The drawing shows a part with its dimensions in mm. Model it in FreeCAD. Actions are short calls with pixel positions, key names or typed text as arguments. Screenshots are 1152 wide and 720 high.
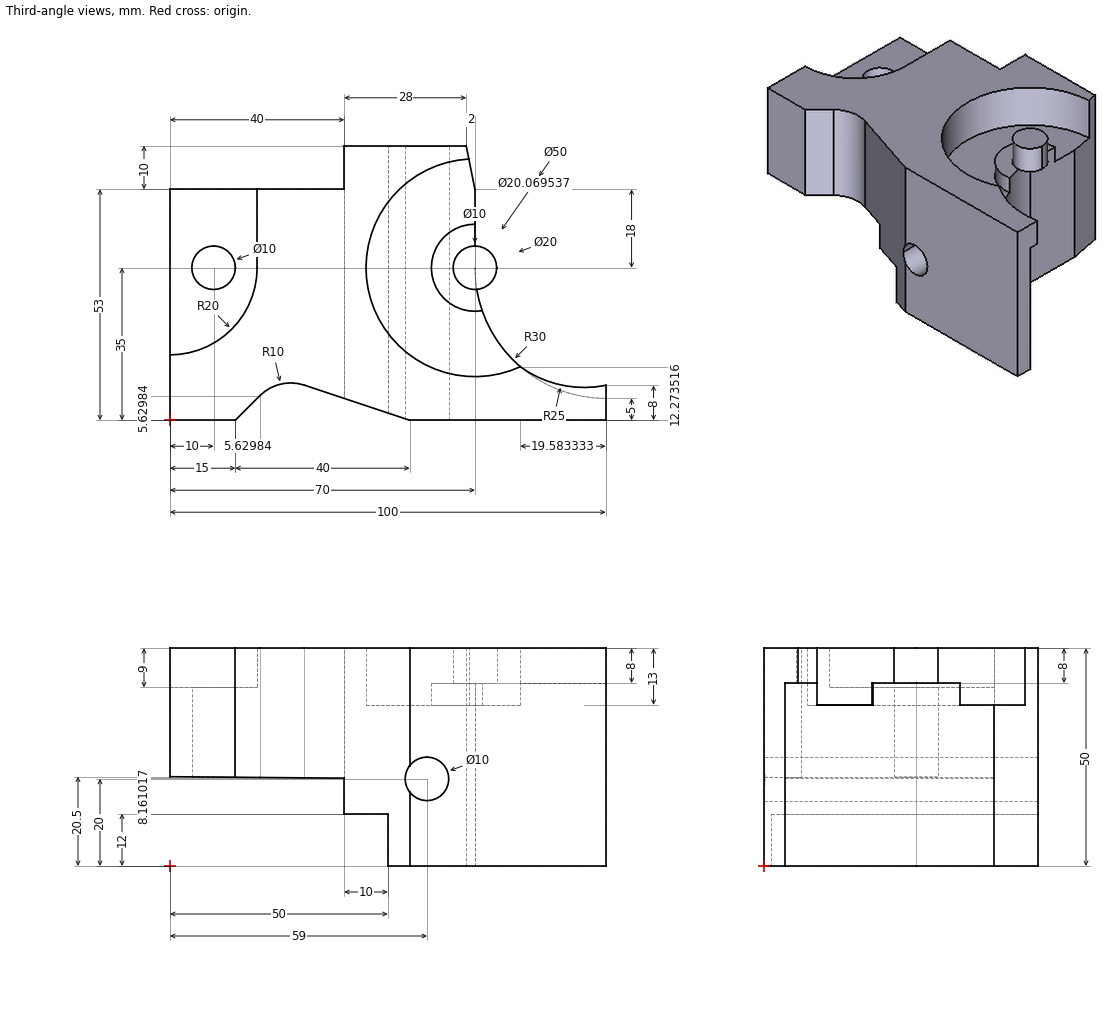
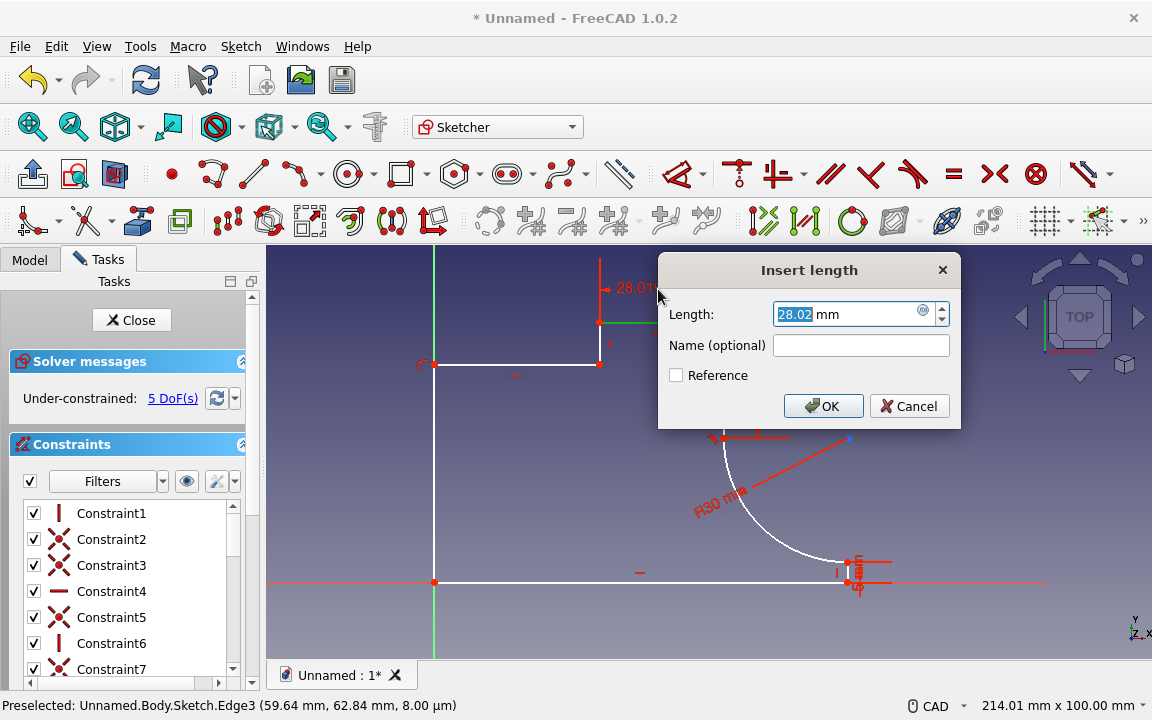
text(28)
key(Return)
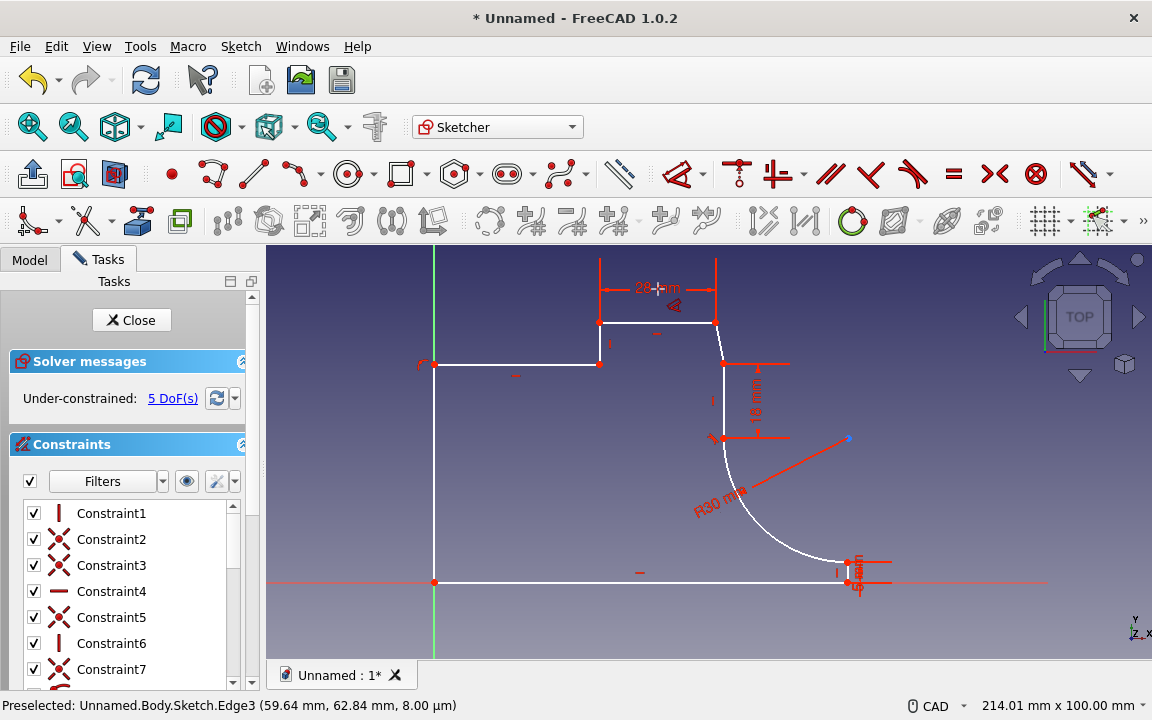
click(600, 335)
click(566, 344)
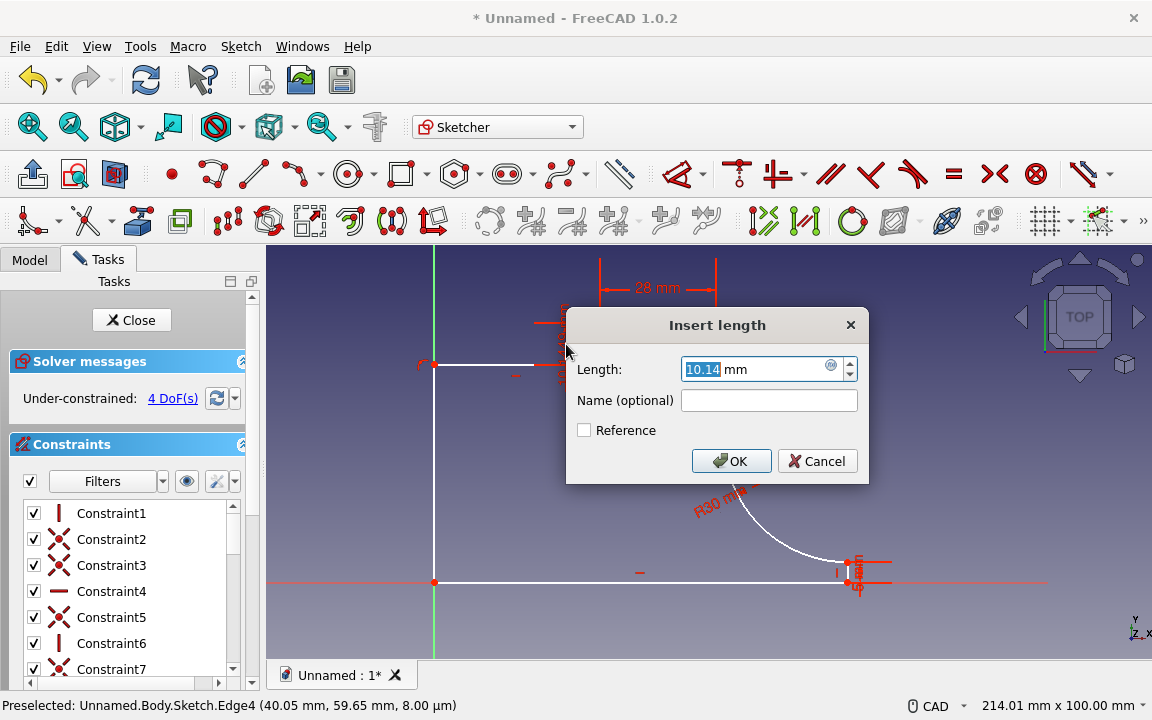
text(10)
key(Return)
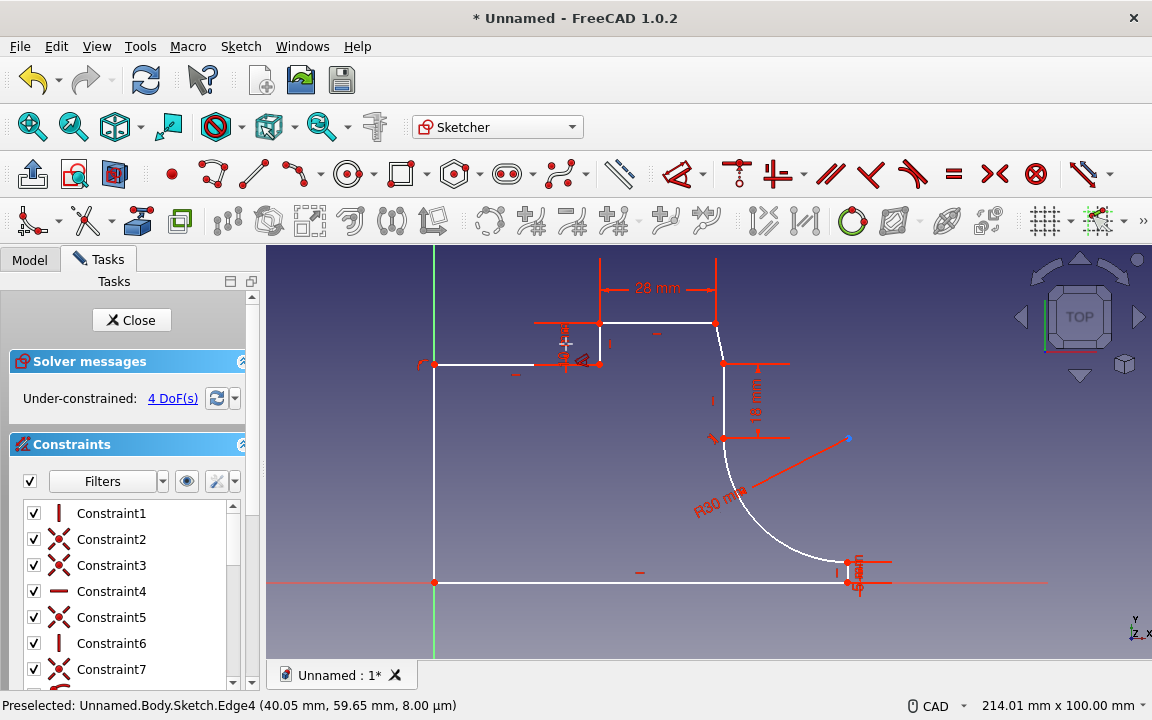
click(550, 364)
click(479, 330)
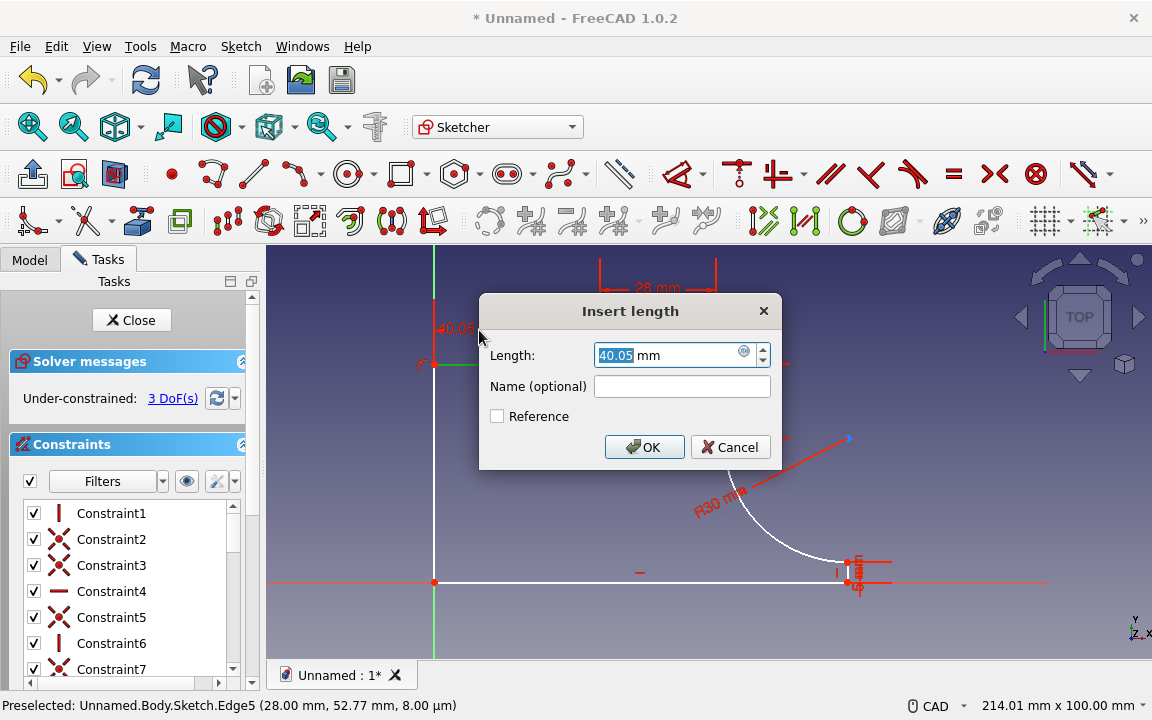
text(40)
key(Return)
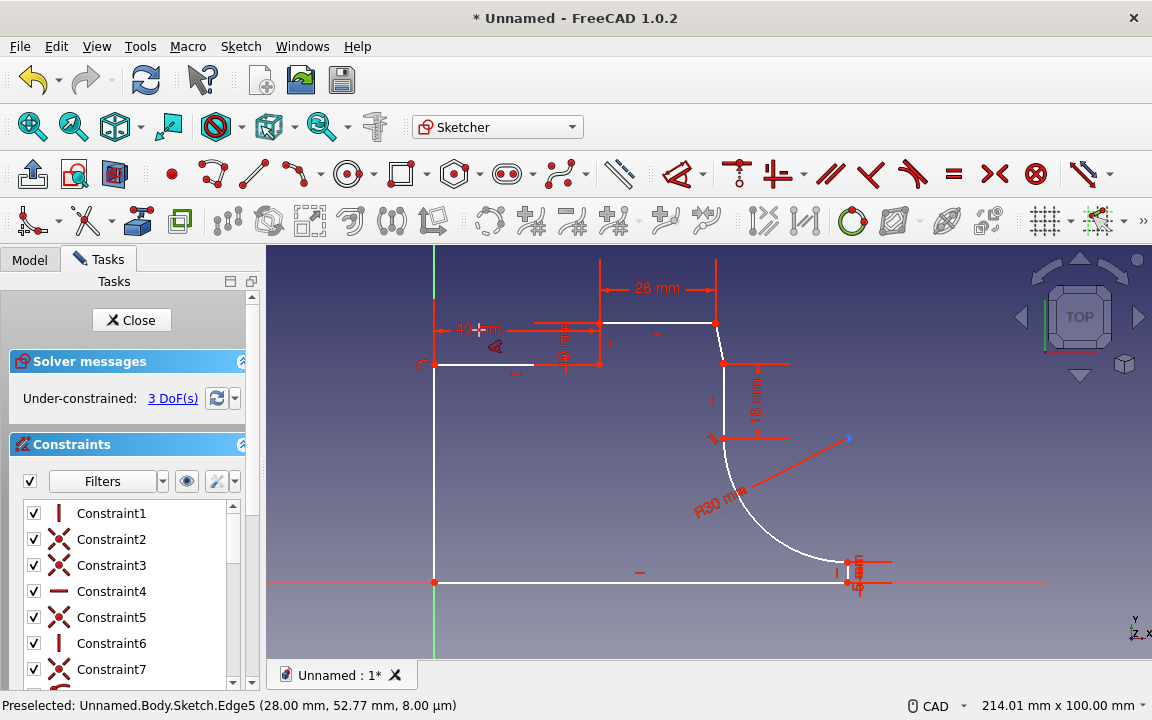
click(434, 430)
click(400, 474)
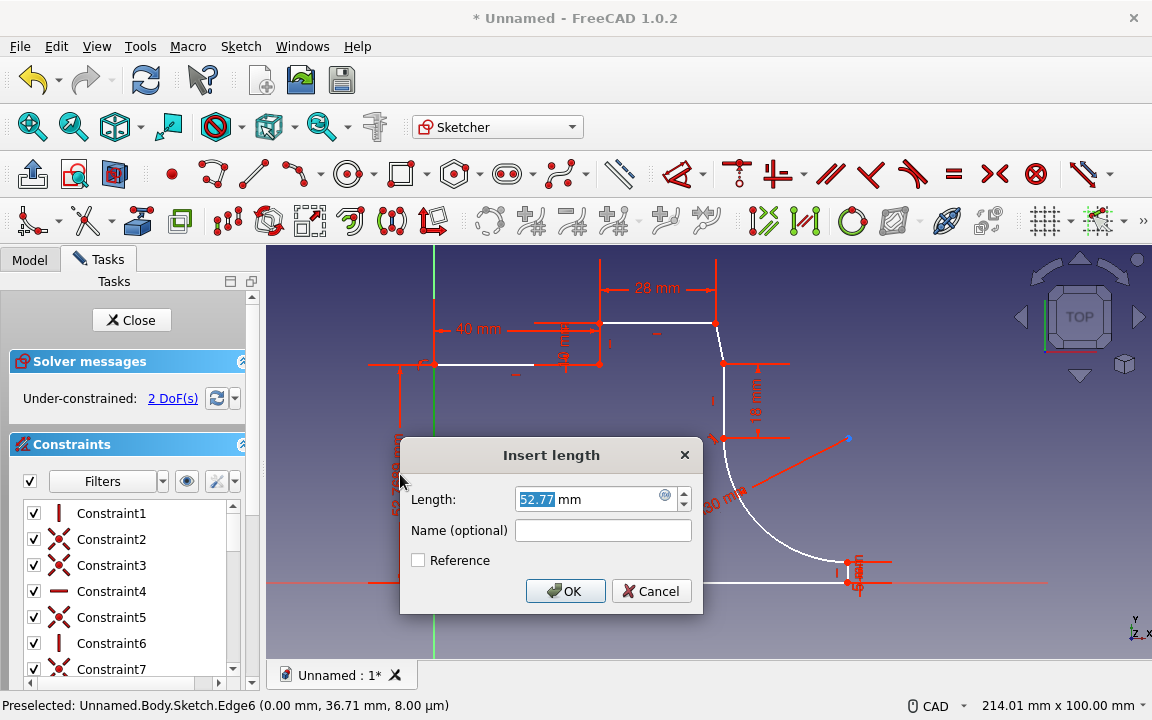
text(53)
key(Return)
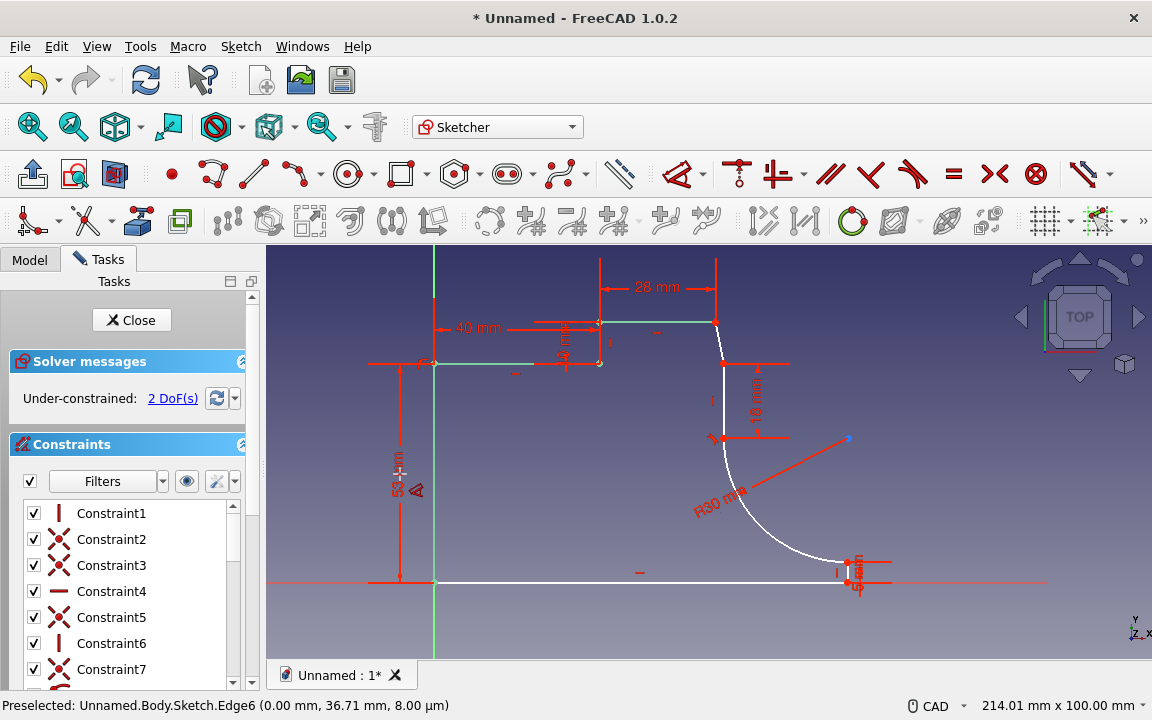
scroll(721, 351, up, 8)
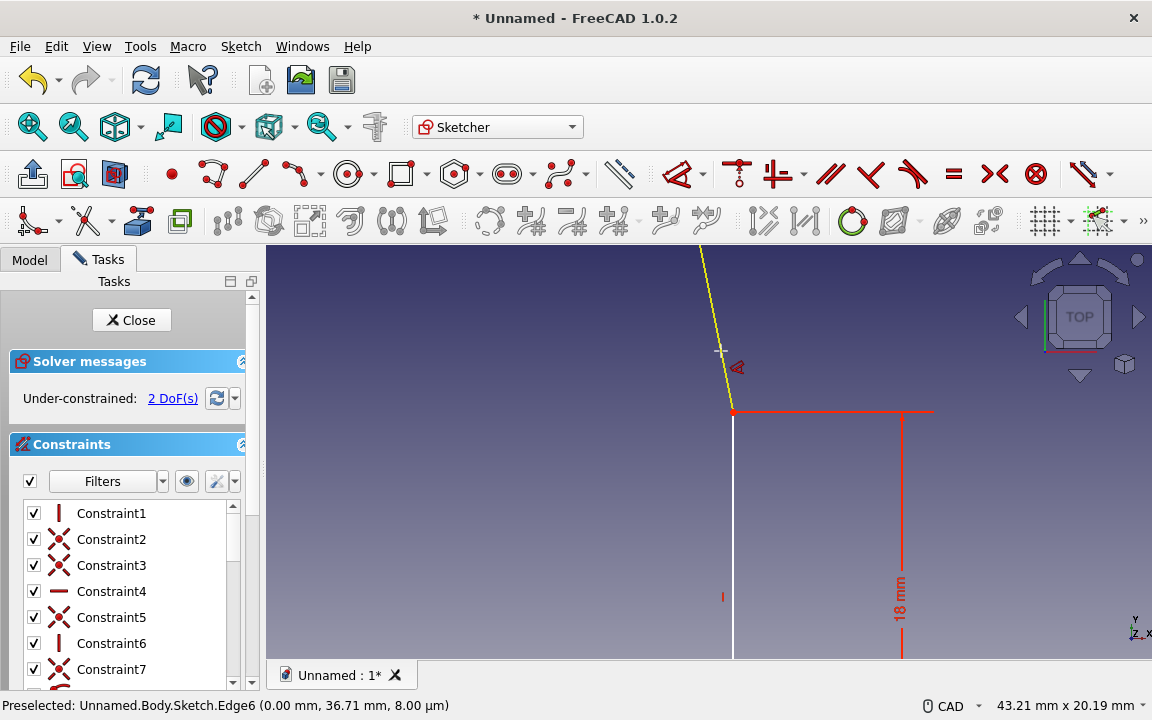
click(721, 351)
click(713, 446)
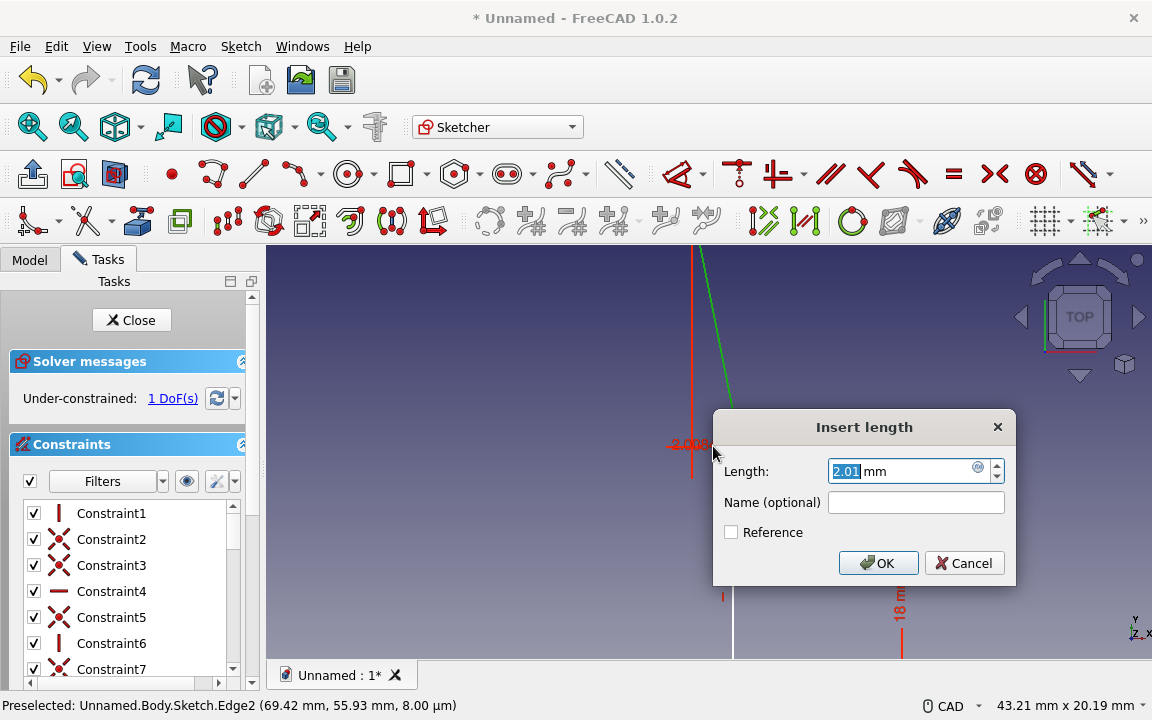
text(2)
key(Return)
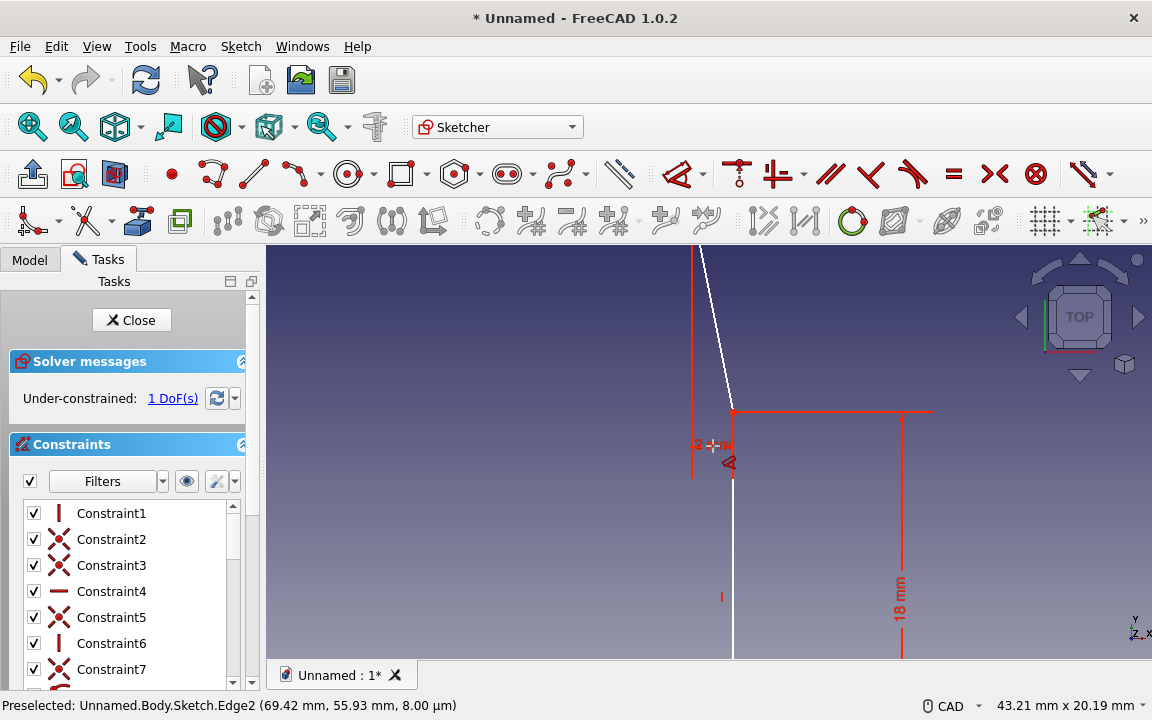
scroll(721, 351, down, 8)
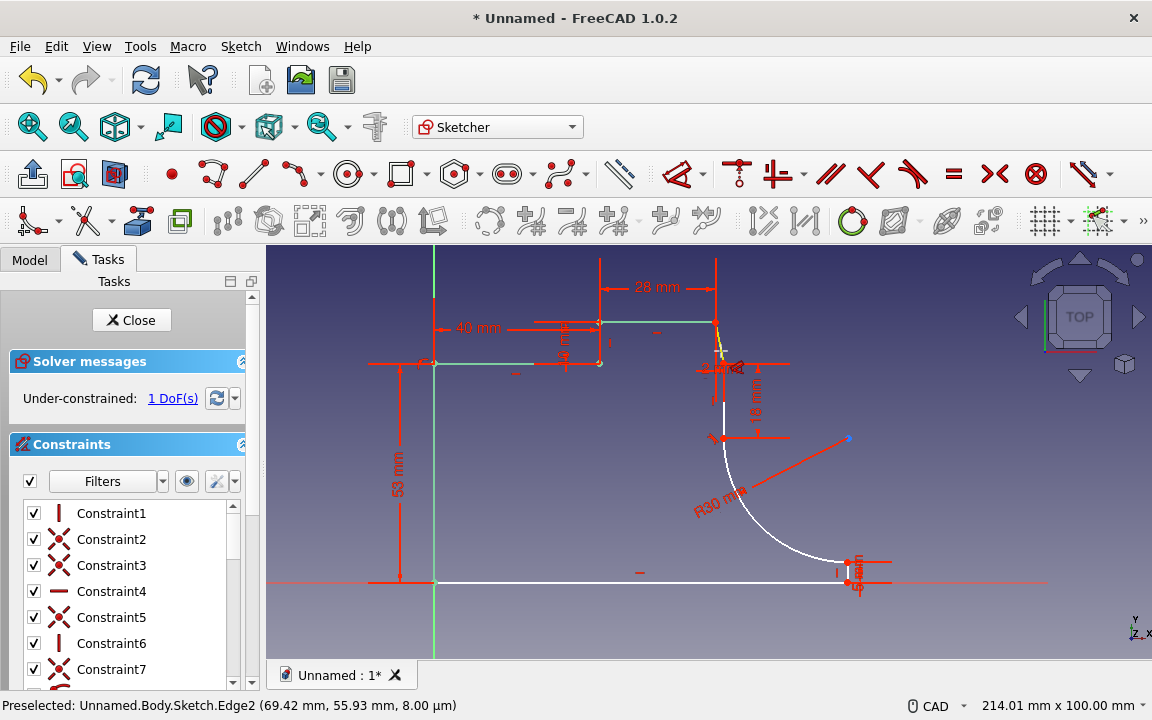
click(558, 583)
click(641, 617)